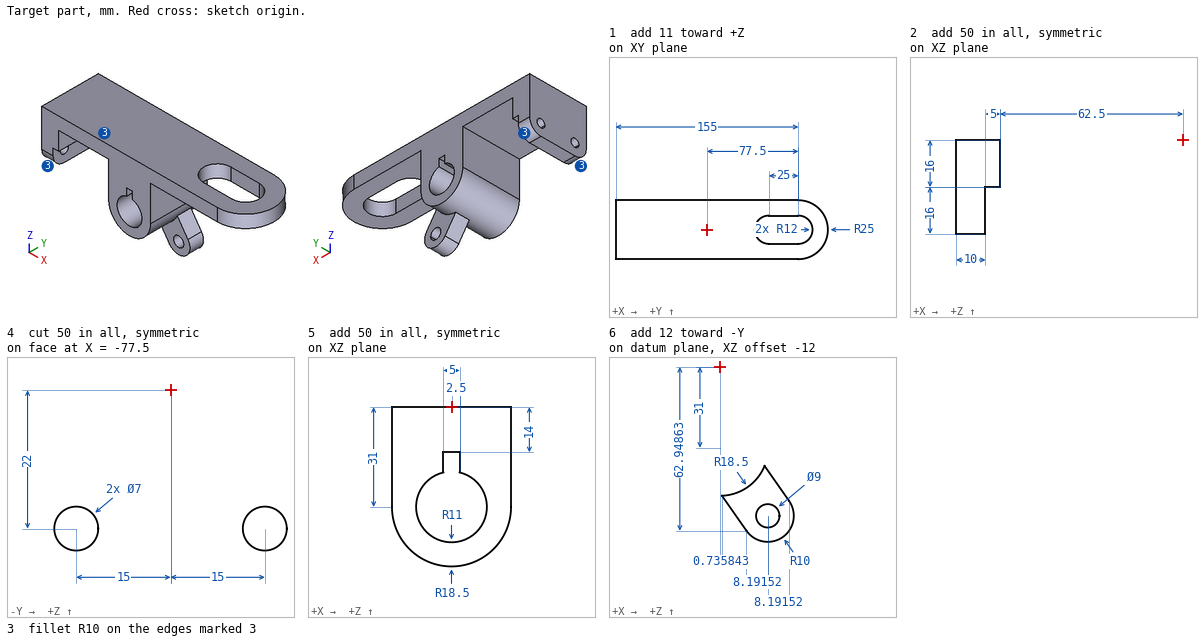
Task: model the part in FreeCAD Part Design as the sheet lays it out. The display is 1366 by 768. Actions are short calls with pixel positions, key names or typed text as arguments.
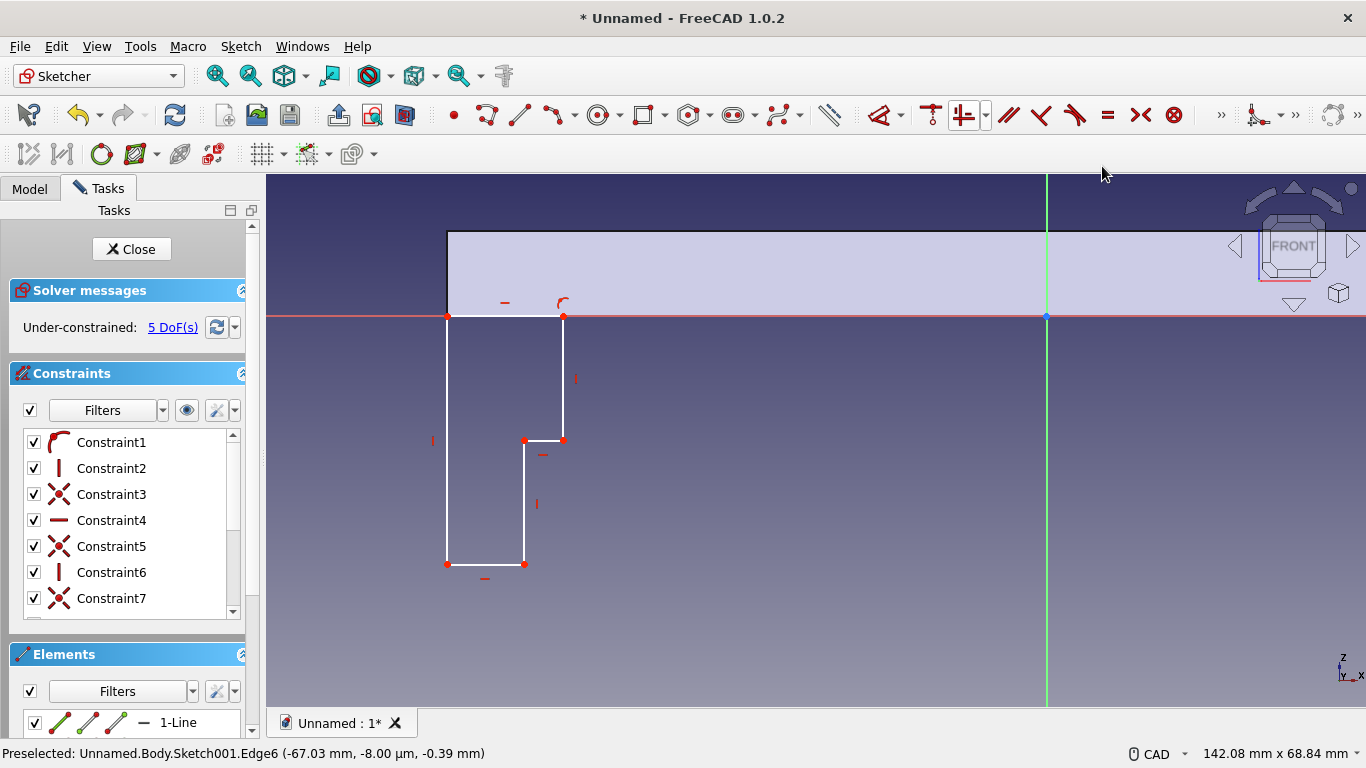
key(d)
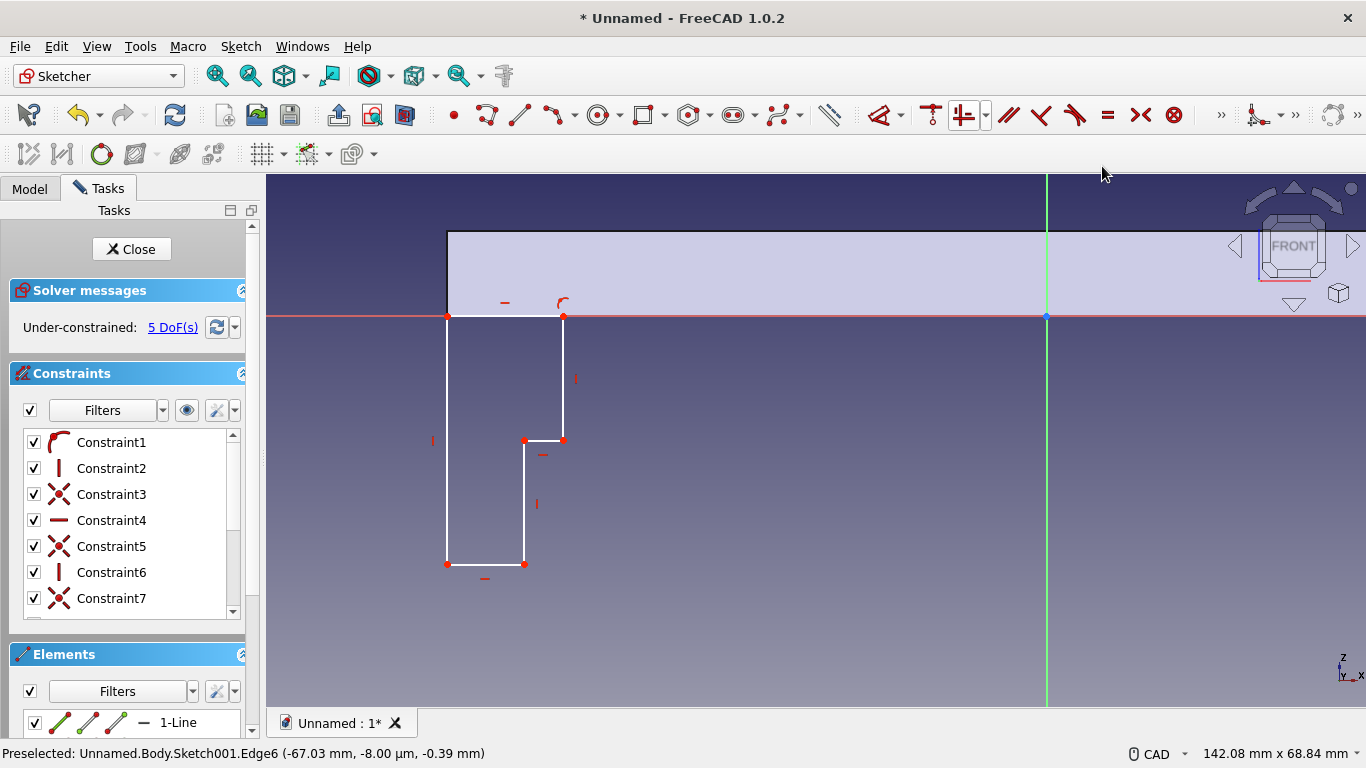
click(551, 441)
click(544, 475)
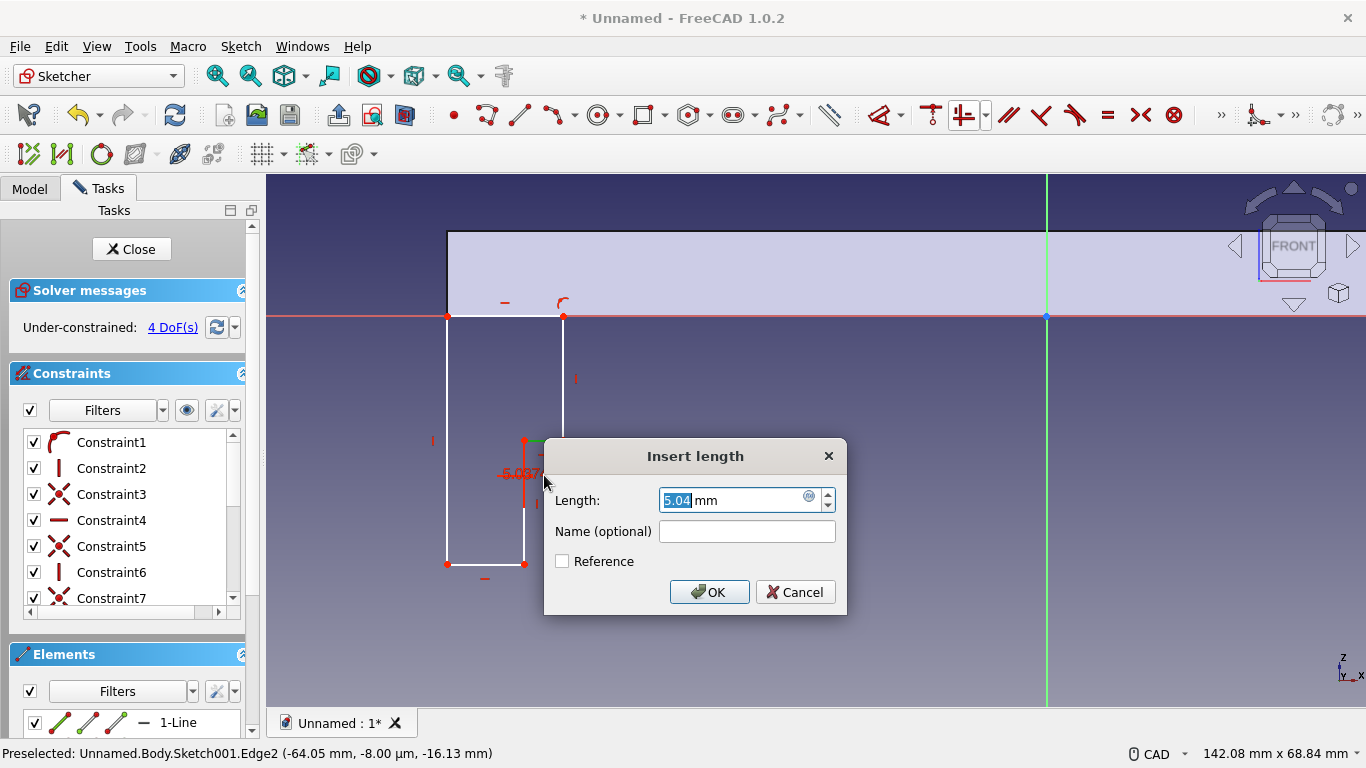
text(5)
key(Return)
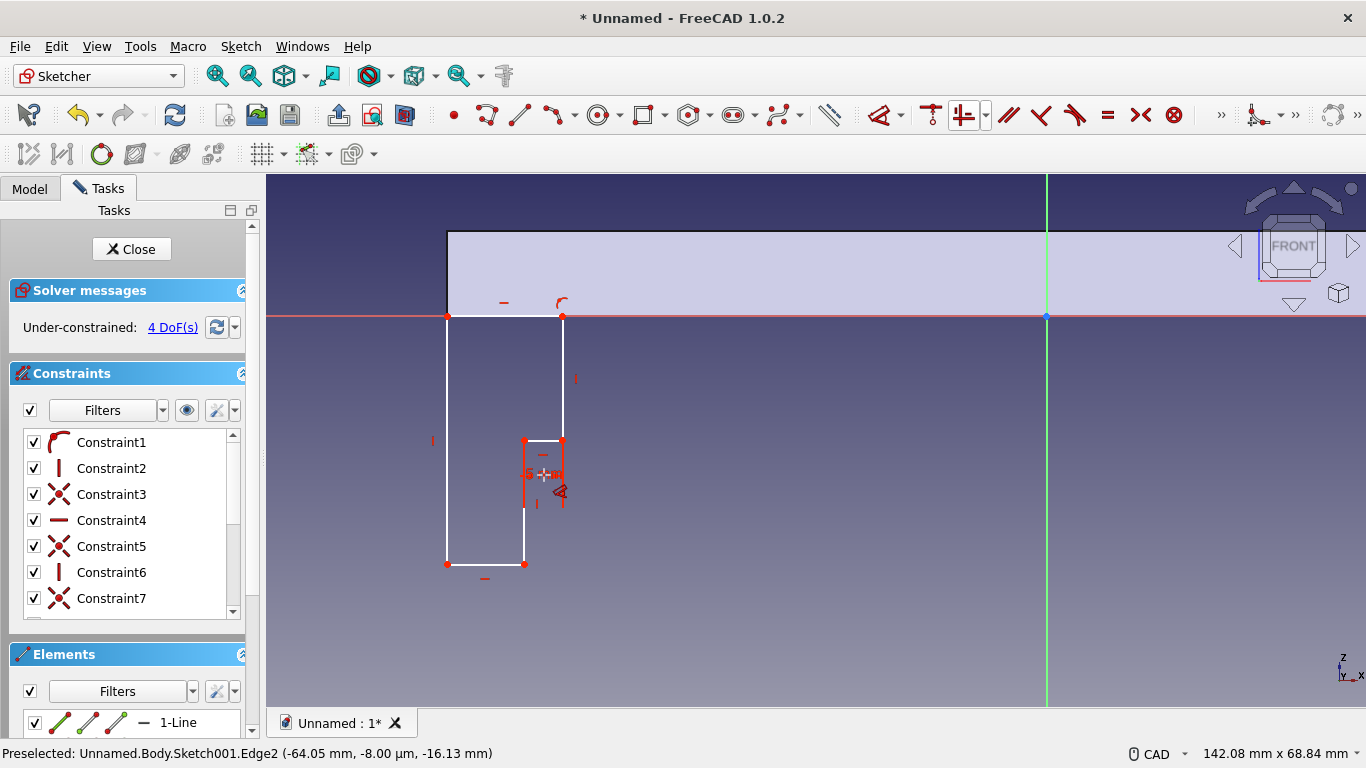
click(563, 354)
click(529, 379)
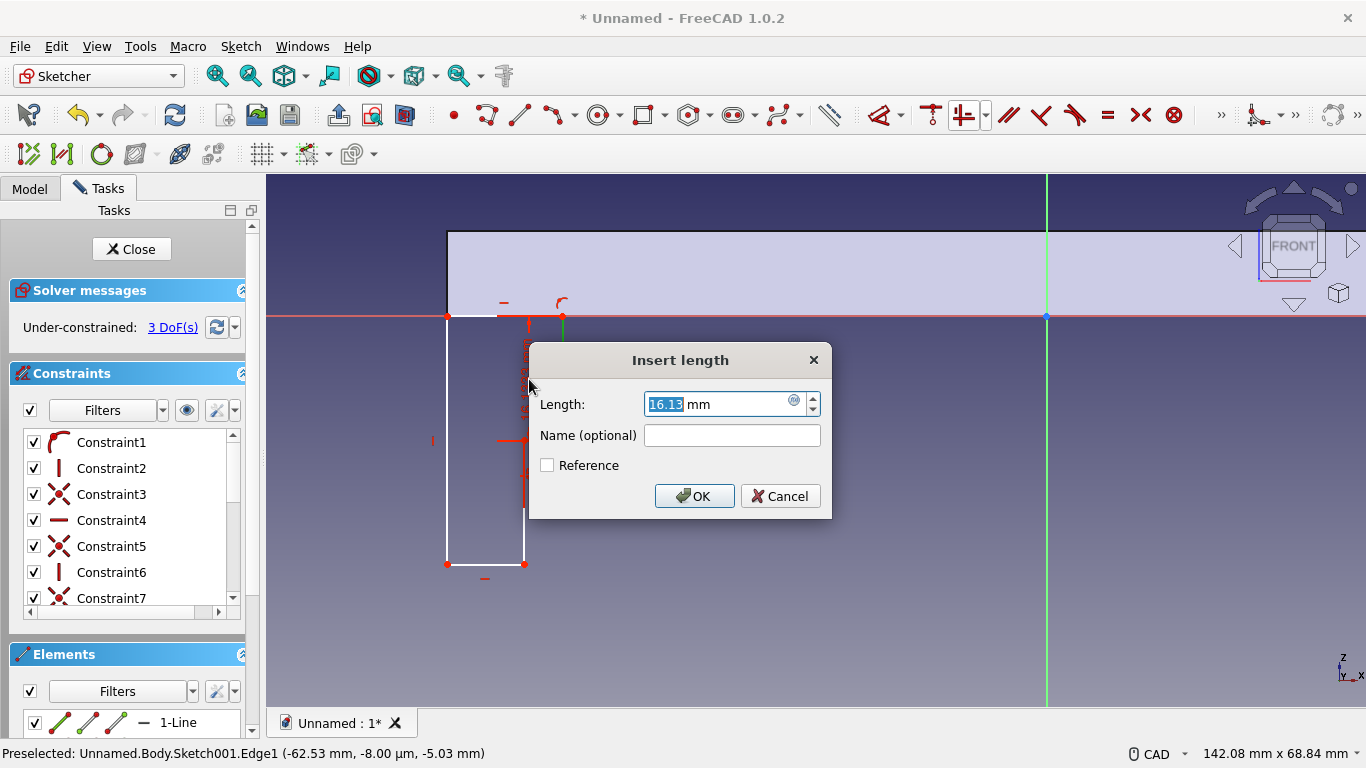
text(16)
key(Return)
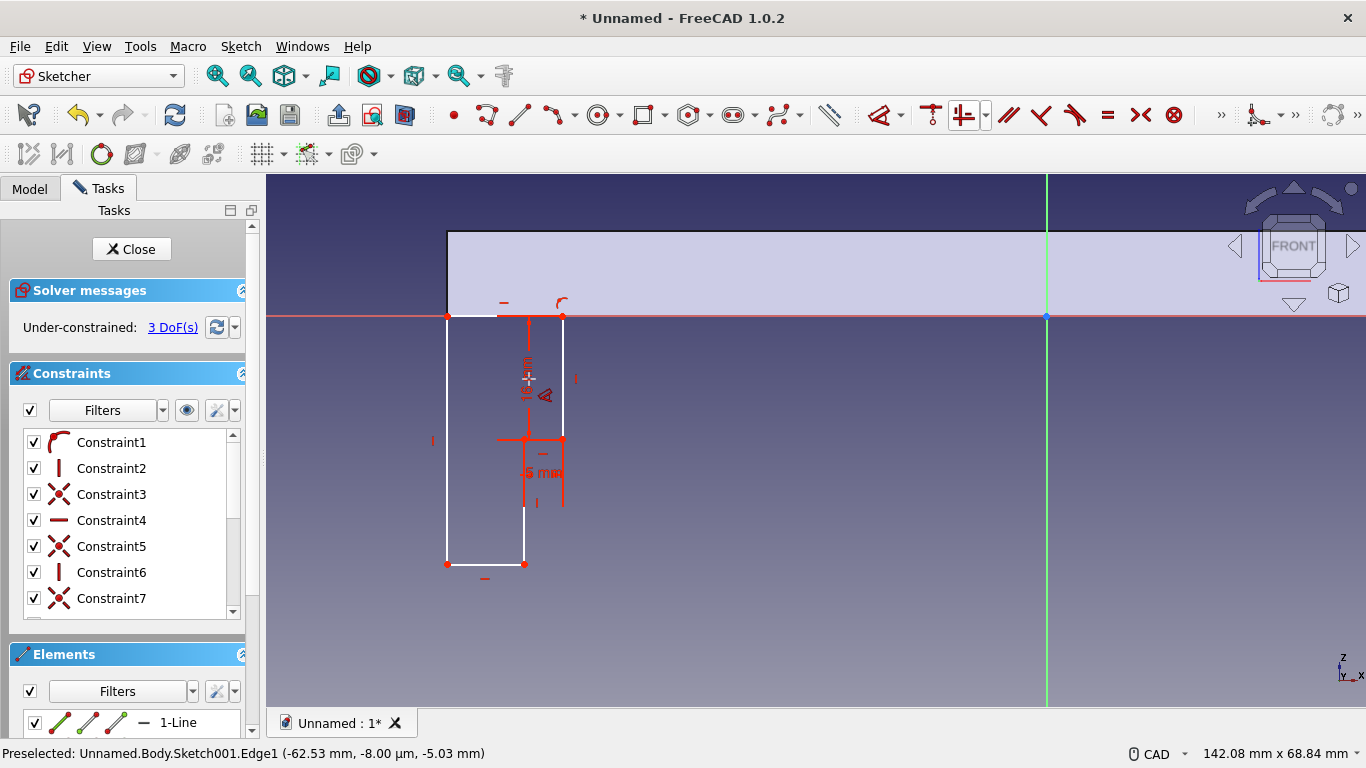
click(524, 477)
click(490, 502)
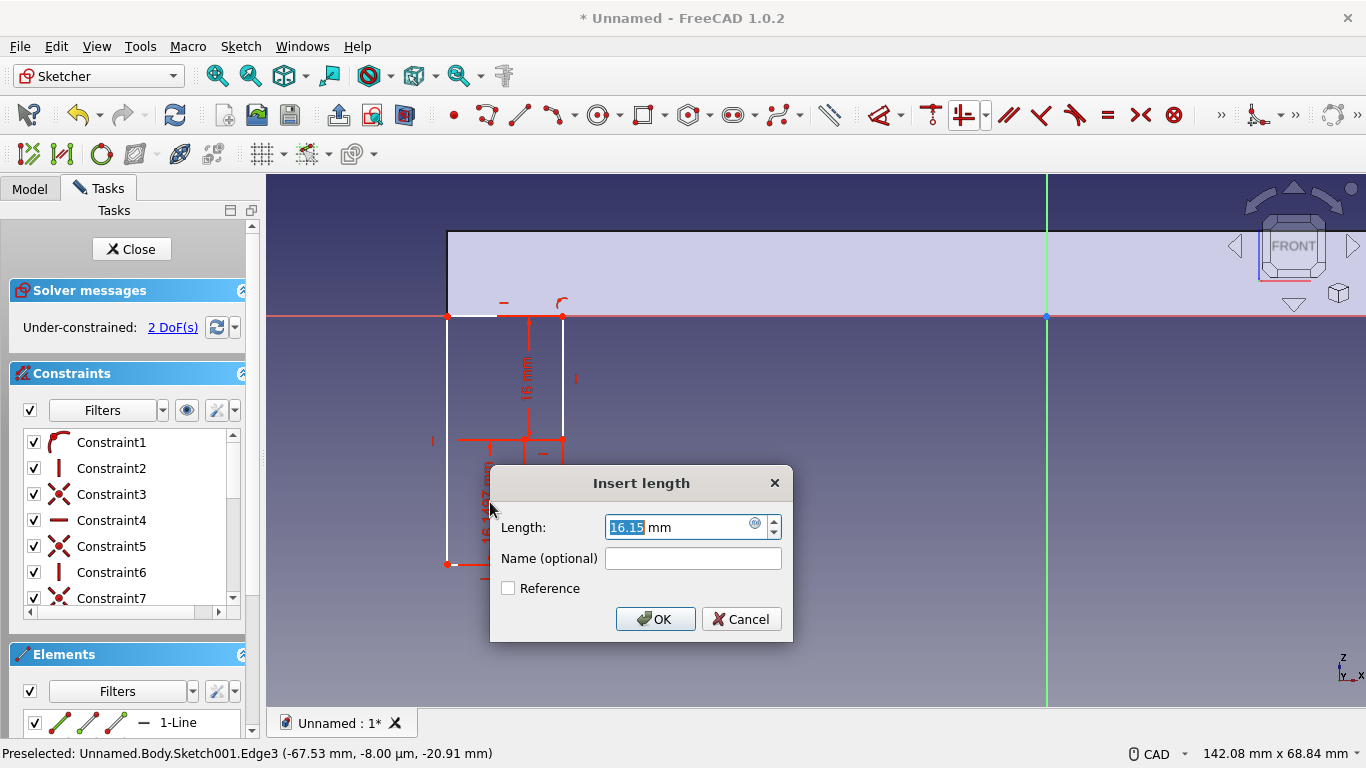
text(16)
key(Return)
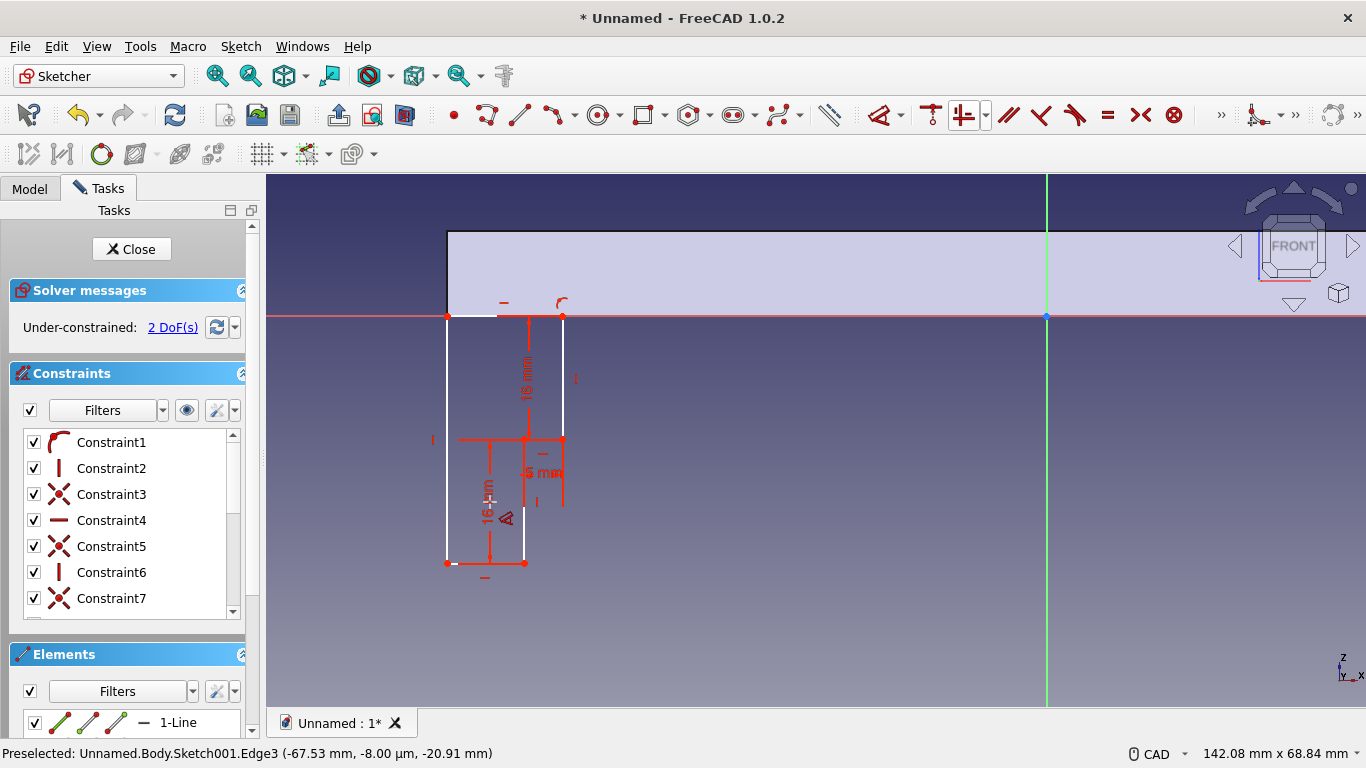
click(501, 564)
click(486, 598)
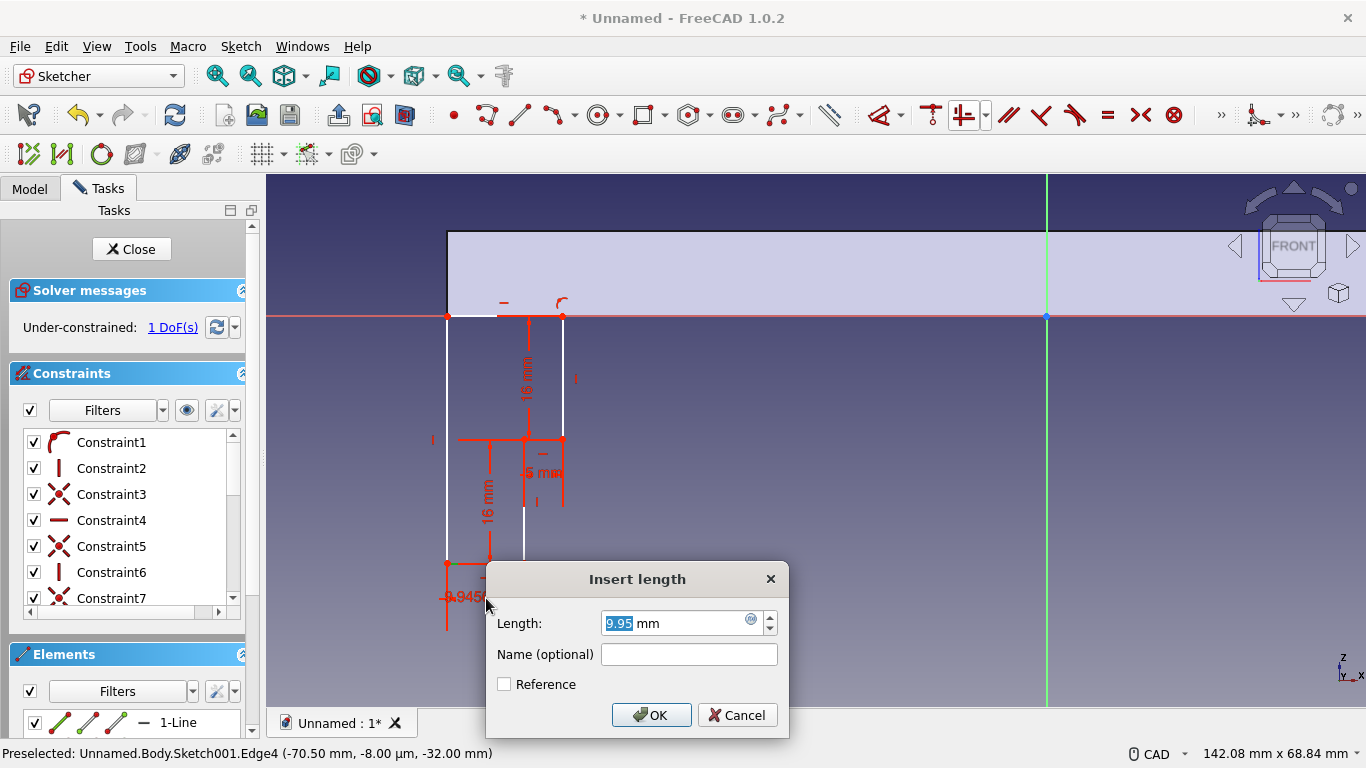
text(10)
key(Return)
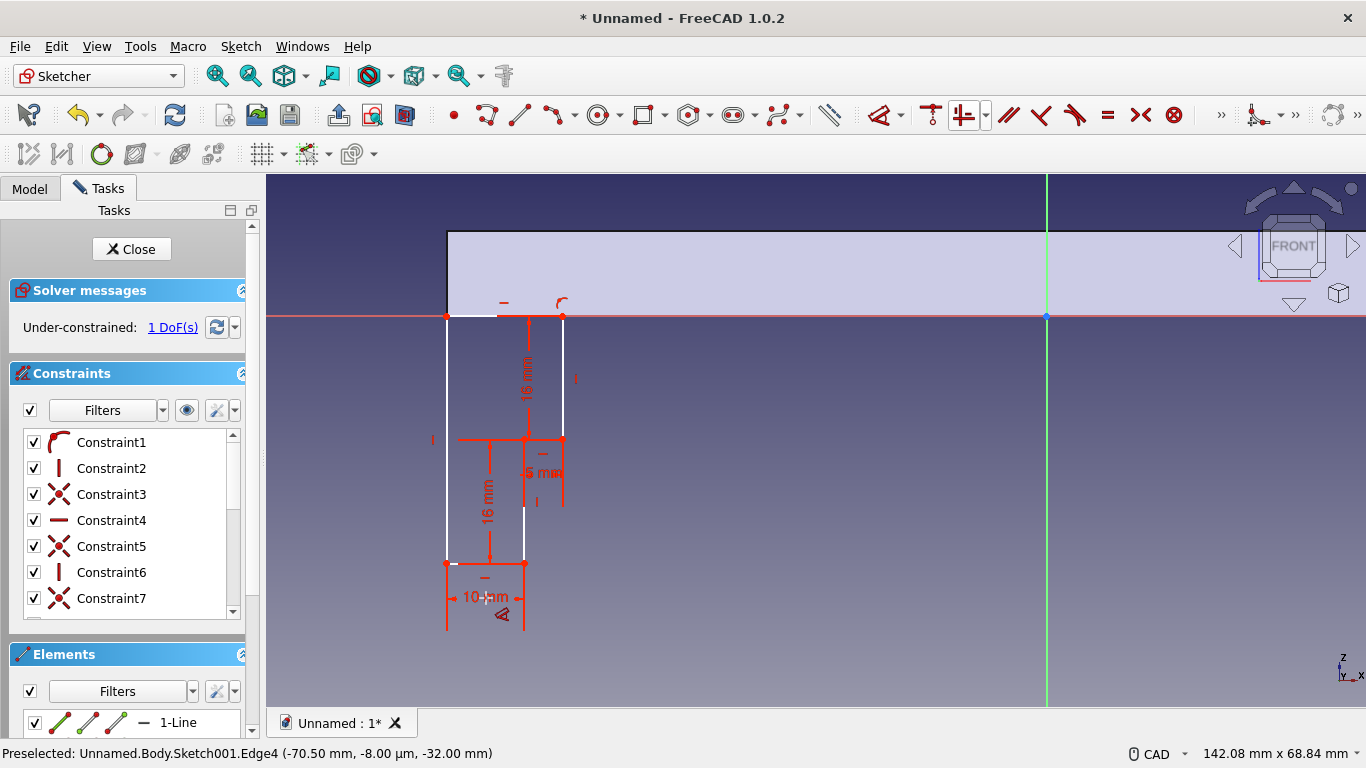
click(563, 316)
click(805, 282)